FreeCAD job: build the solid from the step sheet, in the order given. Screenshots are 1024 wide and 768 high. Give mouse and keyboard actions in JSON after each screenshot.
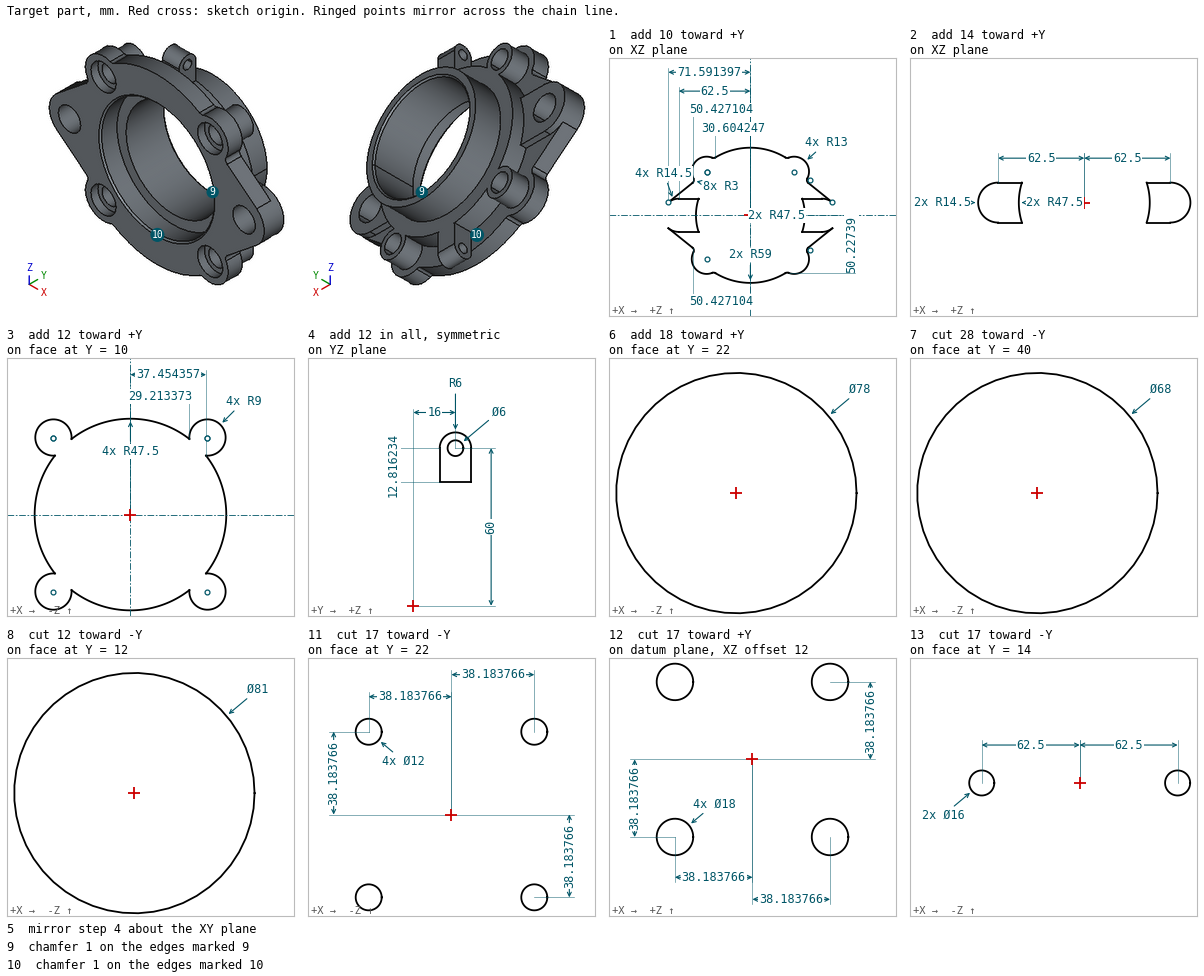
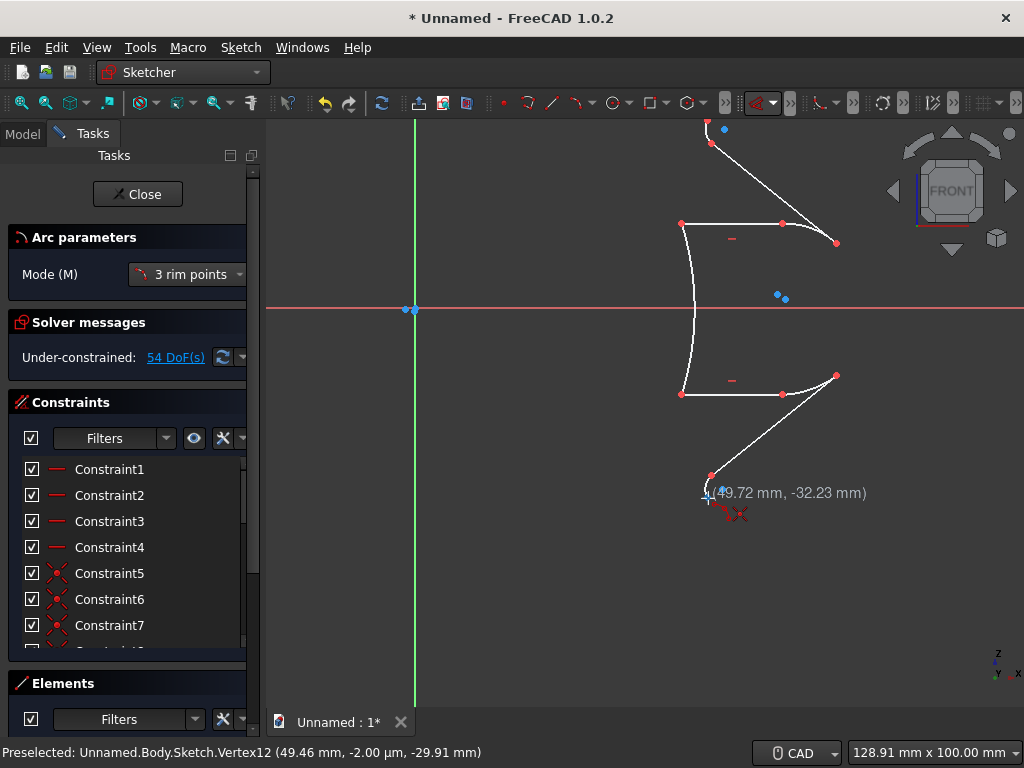
{"action": "left_click", "coordinate": [708, 498]}
{"action": "left_click", "coordinate": [611, 604]}
{"action": "left_click", "coordinate": [697, 584]}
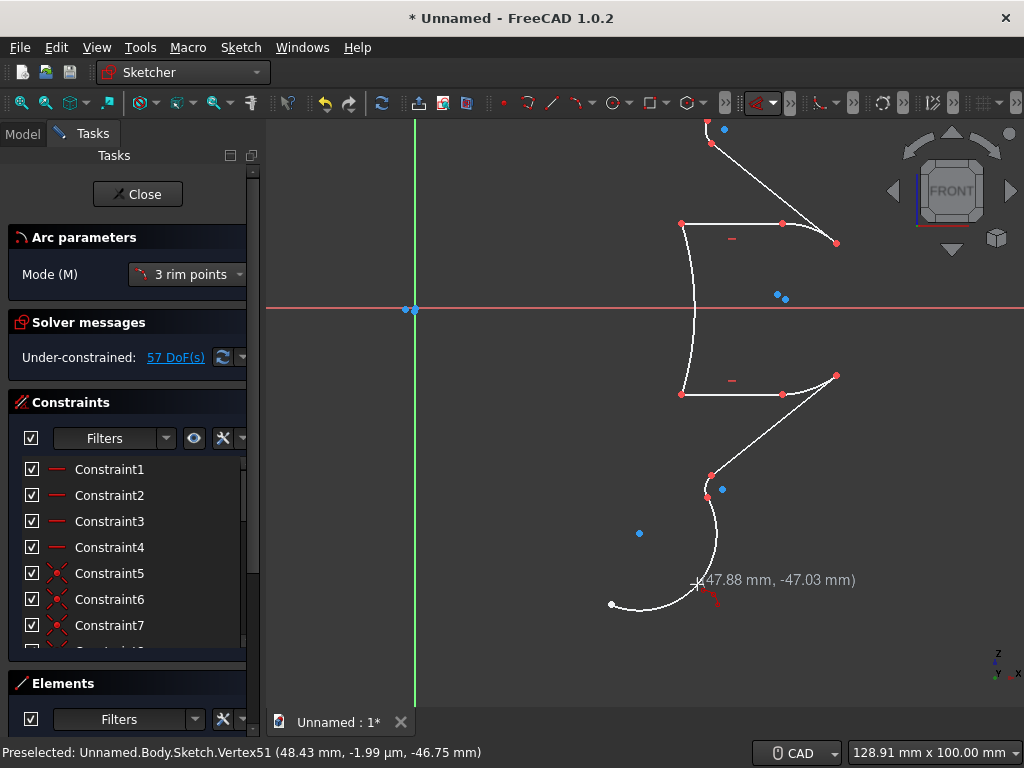
{"action": "left_click", "coordinate": [611, 605]}
{"action": "left_click", "coordinate": [595, 605]}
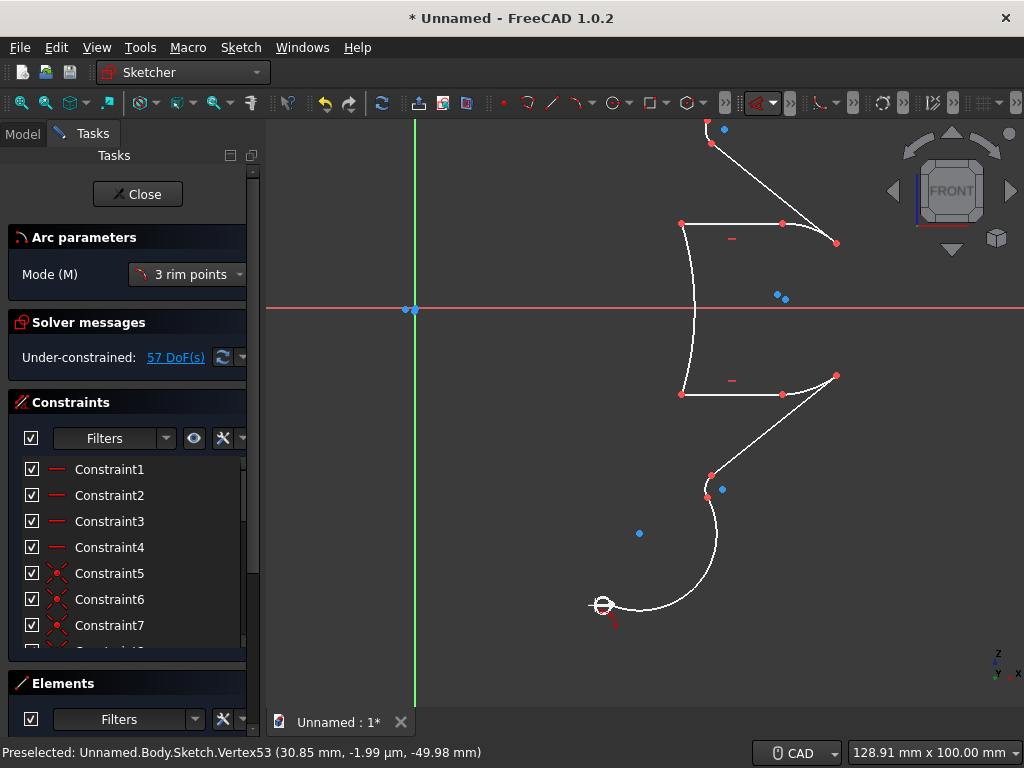
{"action": "scroll", "coordinate": [603, 603], "scroll_direction": "up", "scroll_amount": 11}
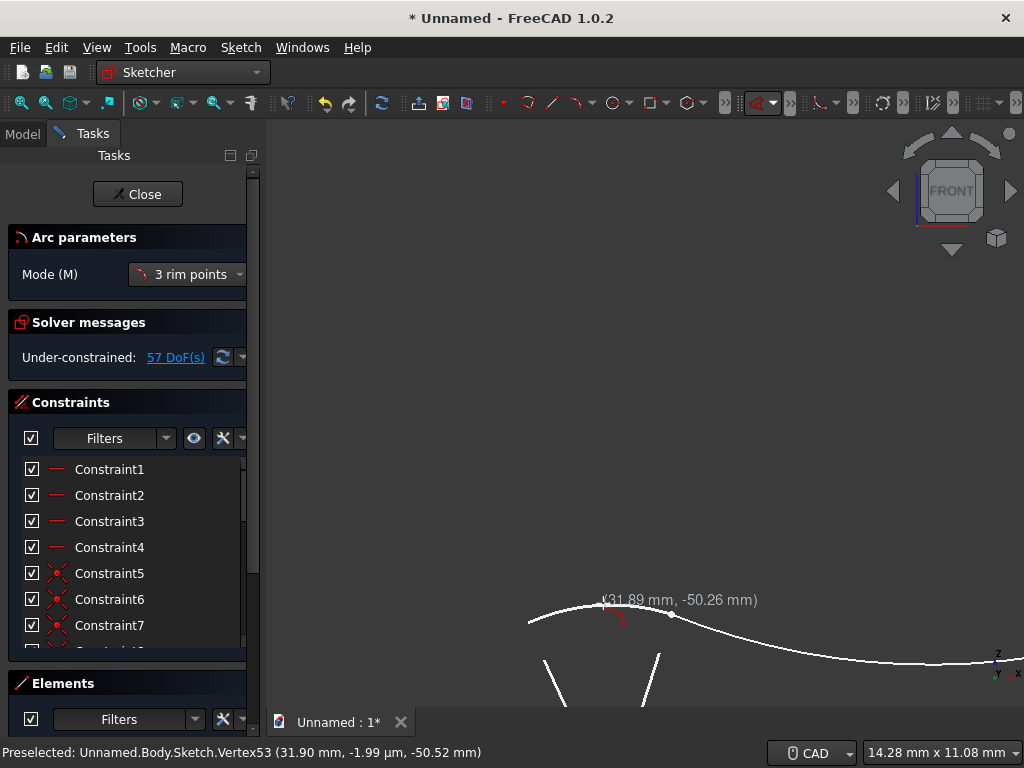
{"action": "left_click", "coordinate": [601, 592]}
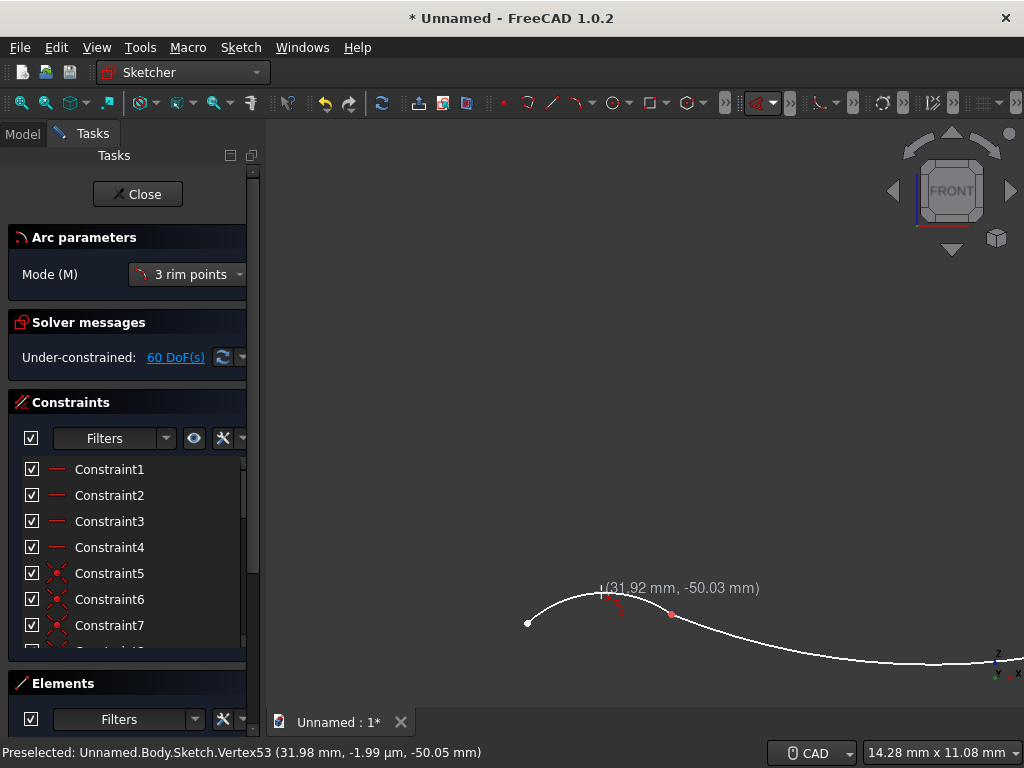
{"action": "scroll", "coordinate": [664, 543], "scroll_direction": "down", "scroll_amount": 15}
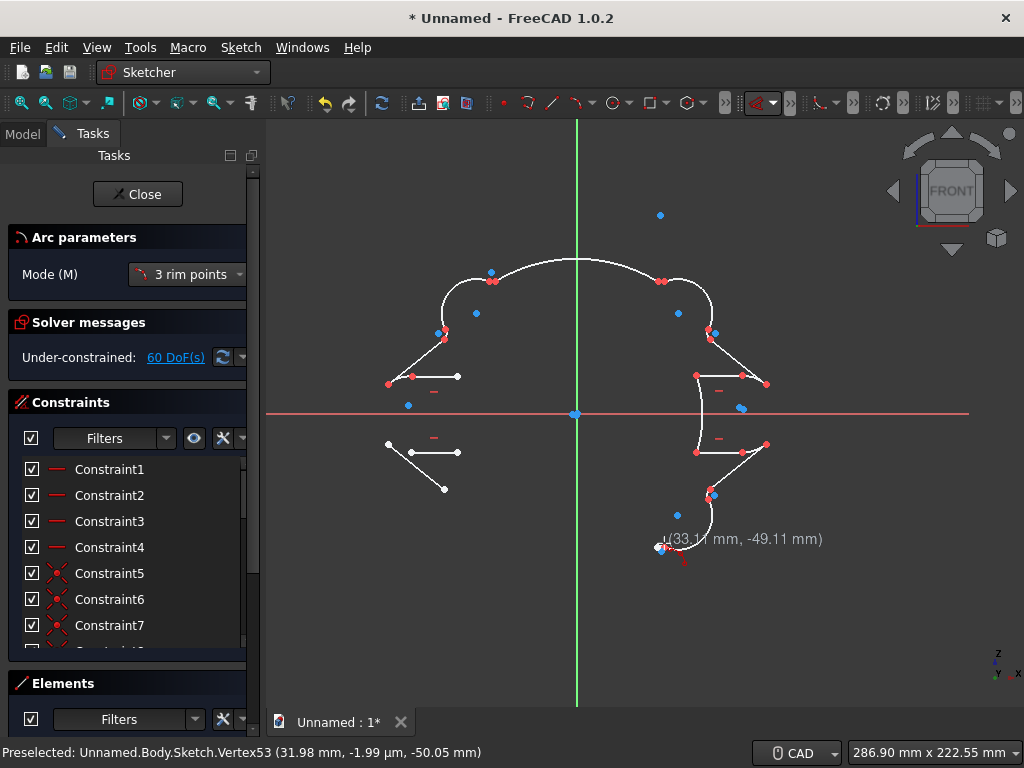
{"action": "scroll", "coordinate": [658, 547], "scroll_direction": "up", "scroll_amount": 5}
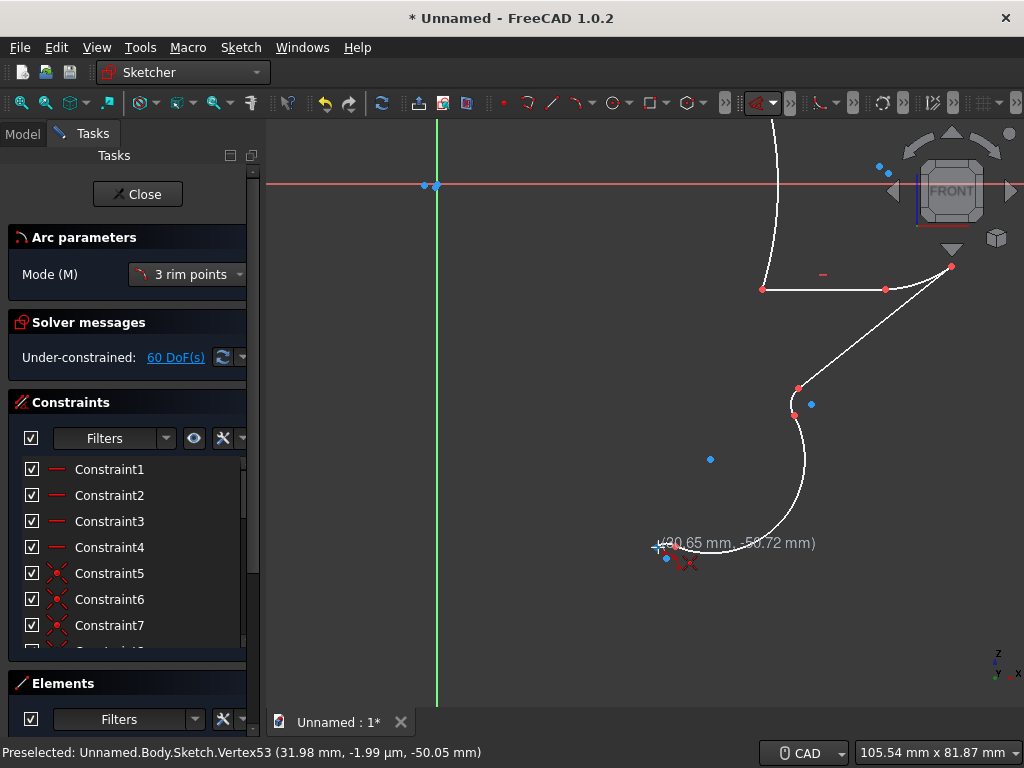
{"action": "left_click", "coordinate": [656, 548]}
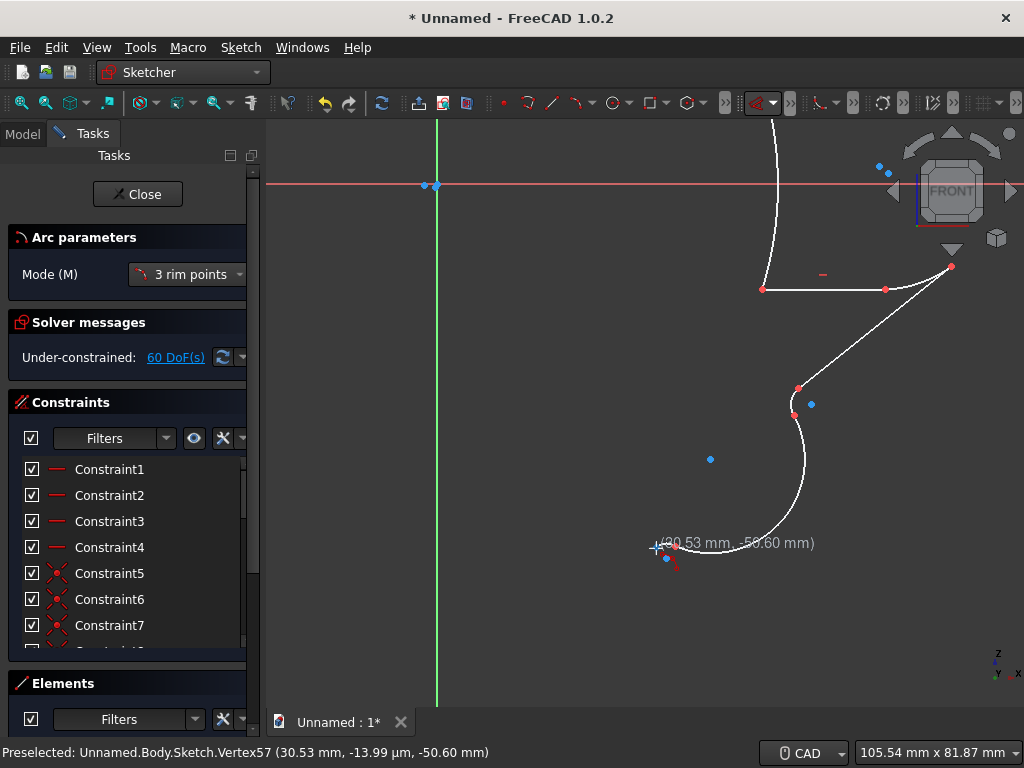
{"action": "scroll", "coordinate": [658, 546], "scroll_direction": "down", "scroll_amount": 5}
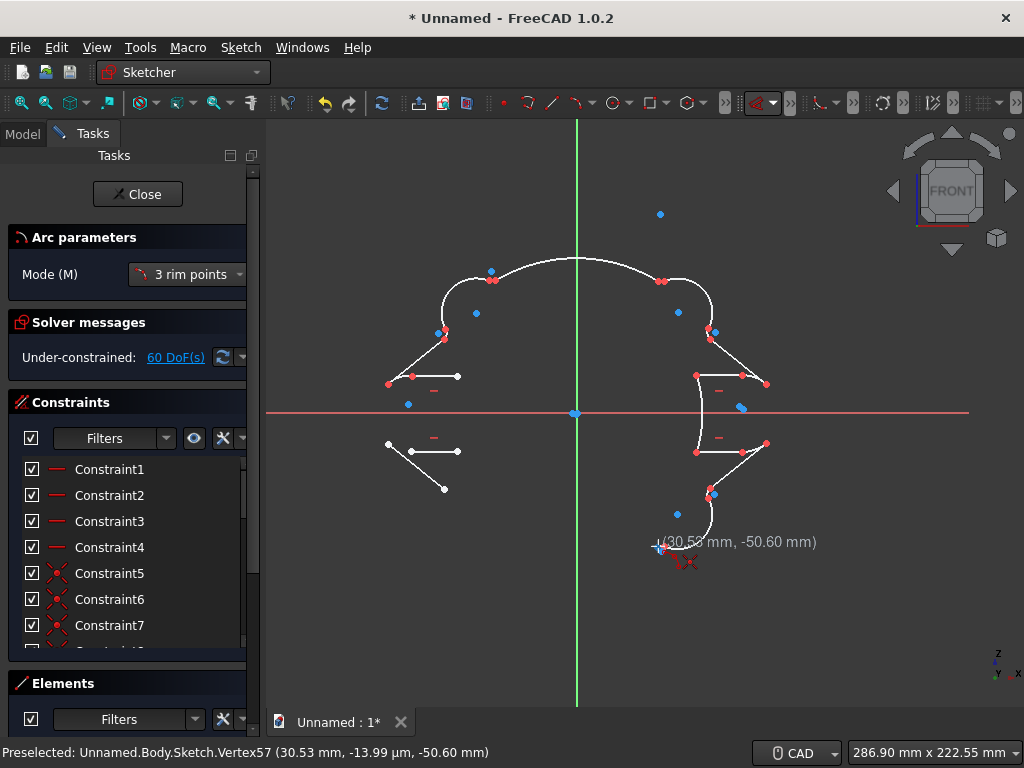
{"action": "left_click", "coordinate": [496, 547]}
{"action": "left_click", "coordinate": [560, 568]}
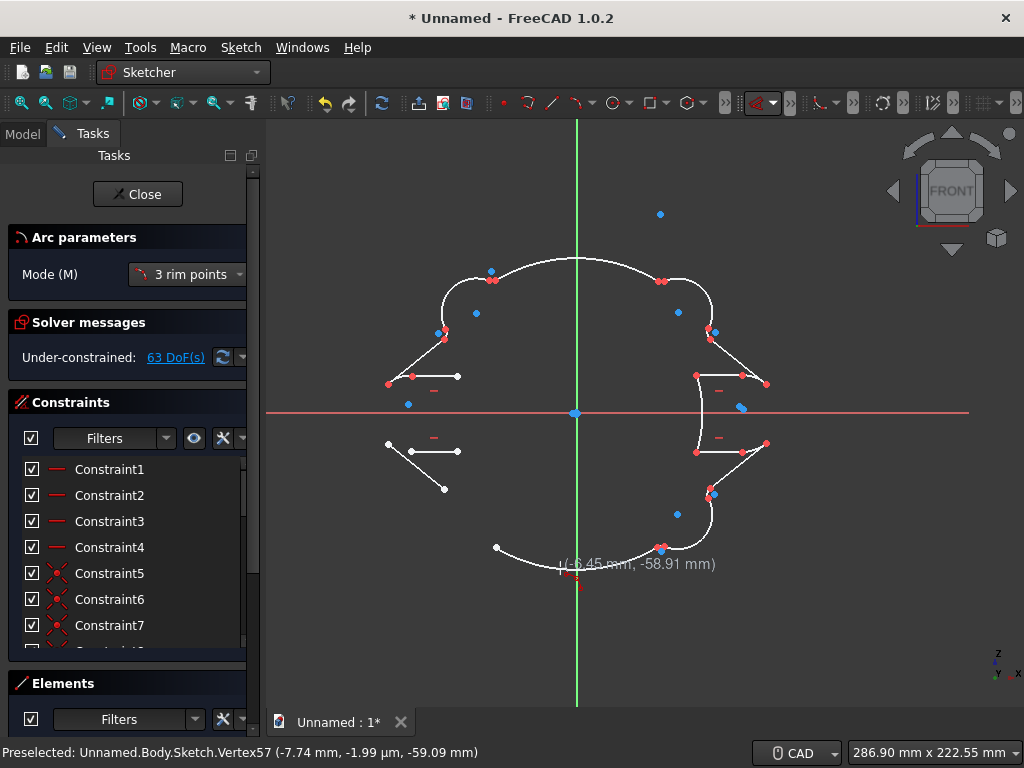
{"action": "left_click", "coordinate": [496, 548]}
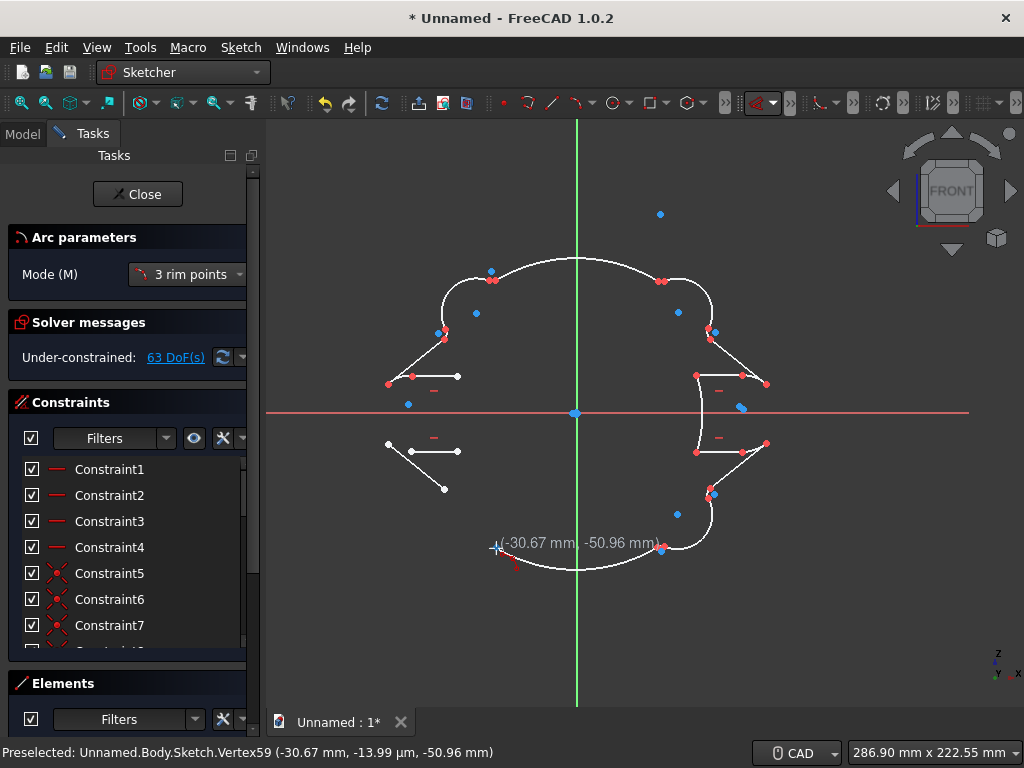
{"action": "scroll", "coordinate": [489, 546], "scroll_direction": "up", "scroll_amount": 5}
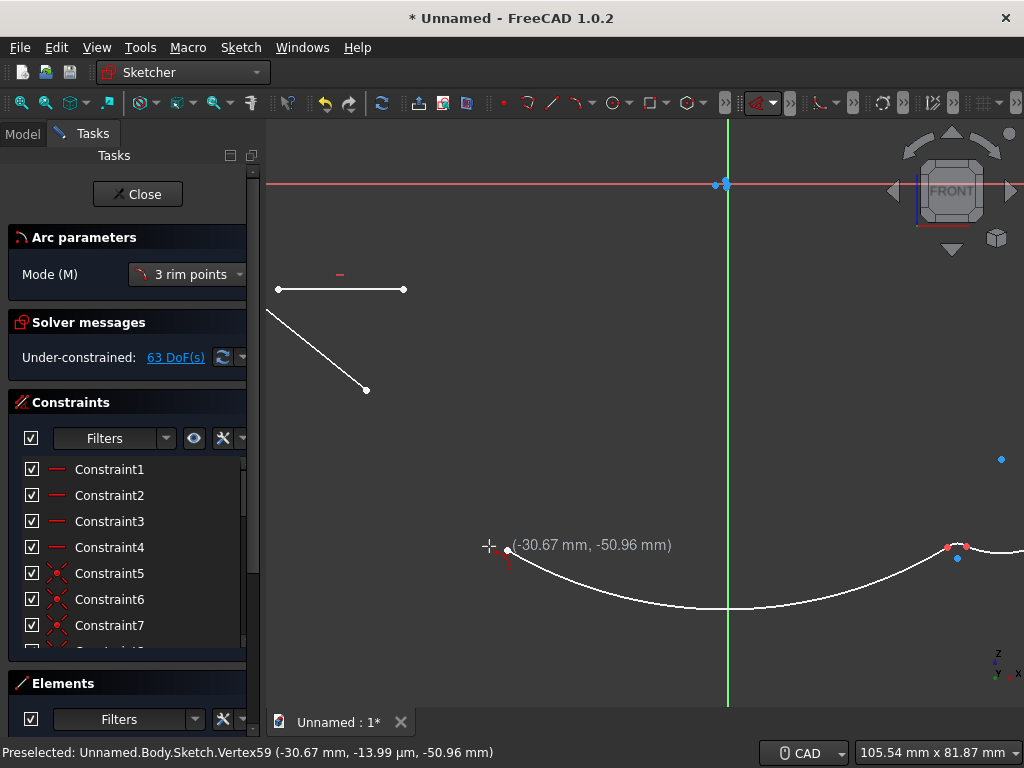
{"action": "left_click", "coordinate": [489, 545]}